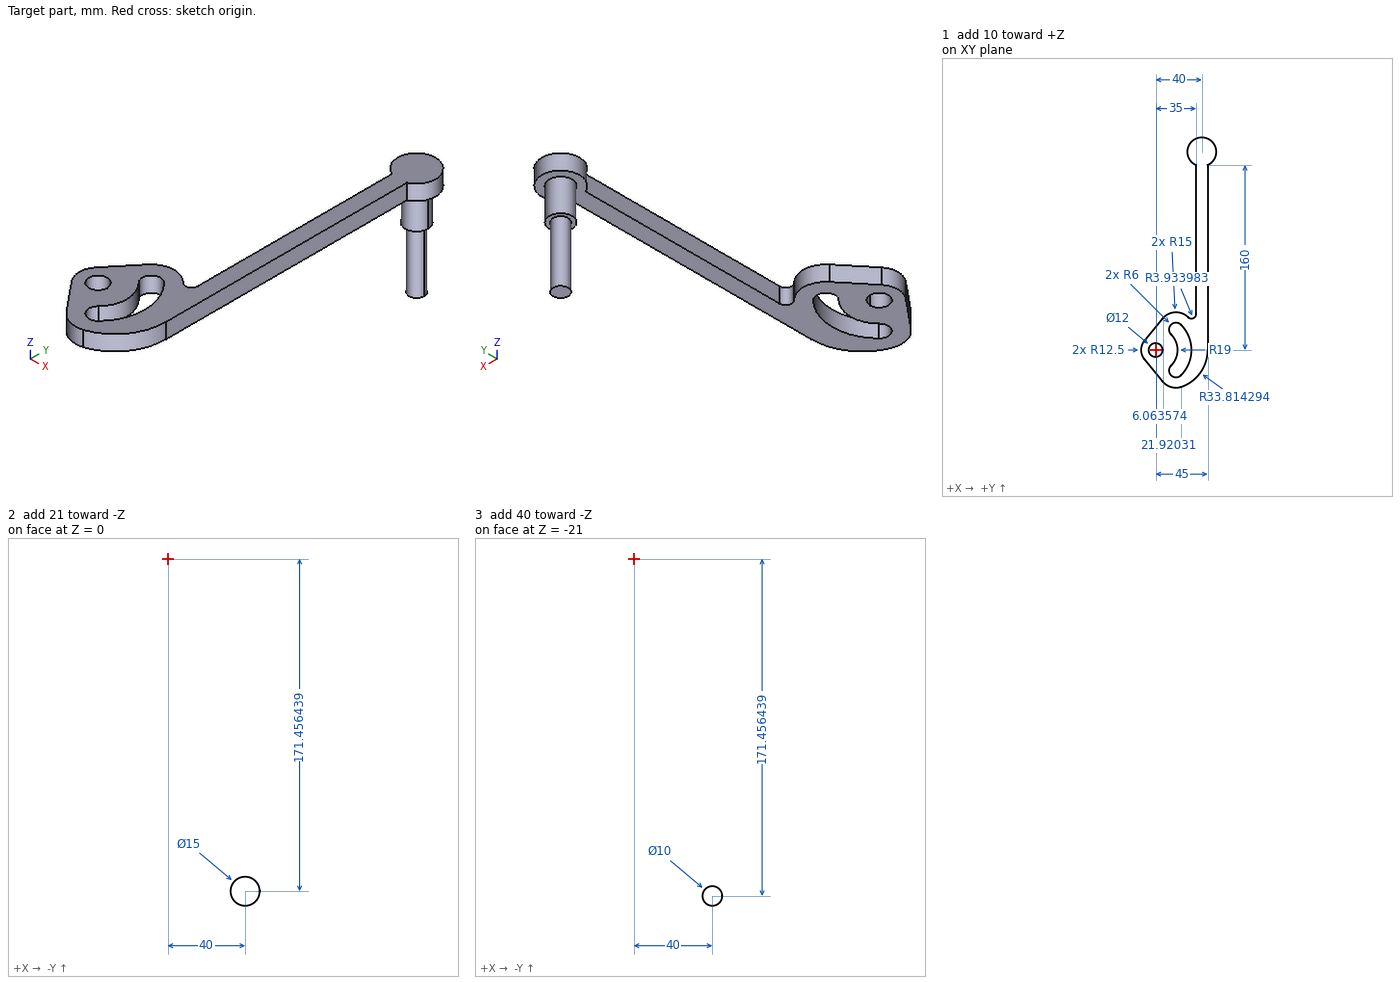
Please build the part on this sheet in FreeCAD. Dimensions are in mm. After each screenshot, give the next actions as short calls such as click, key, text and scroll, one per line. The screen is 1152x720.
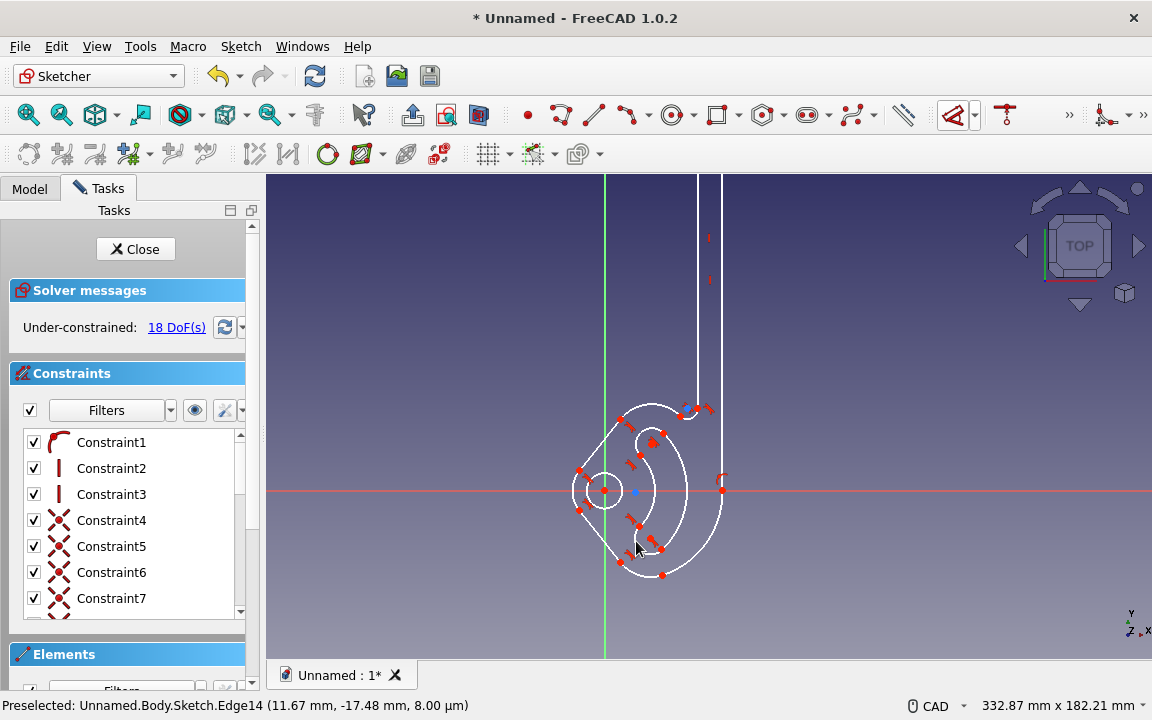
scroll(605, 491, up, 7)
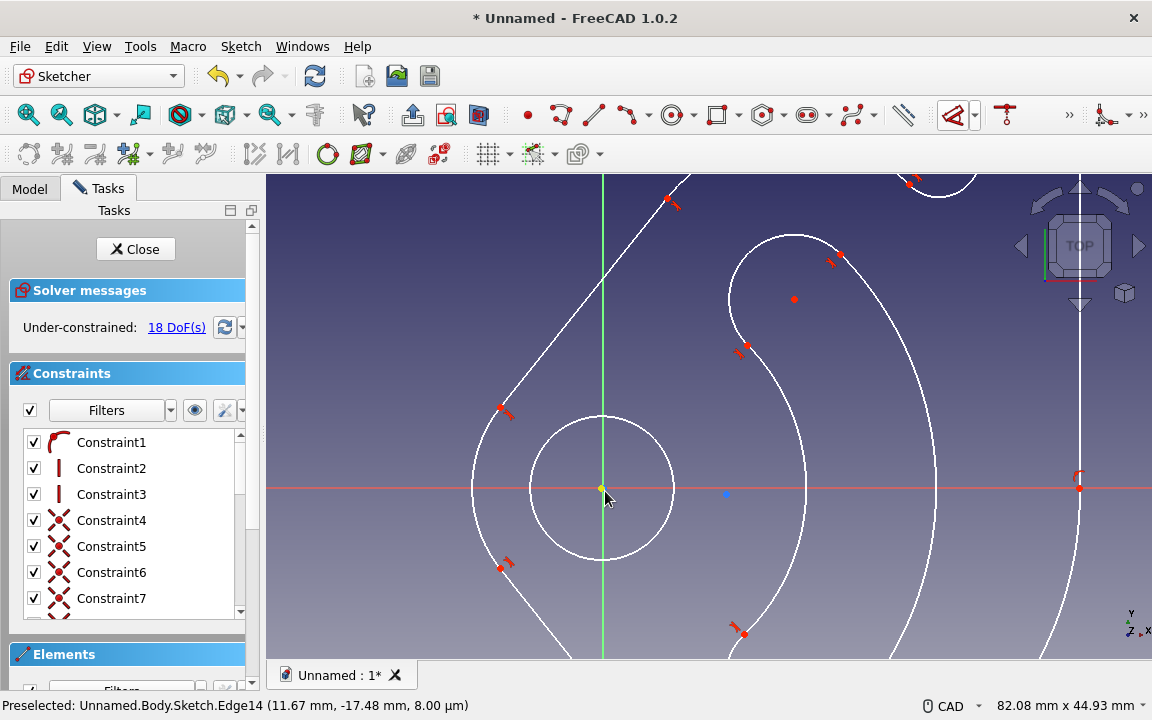
drag(592, 478, 613, 498)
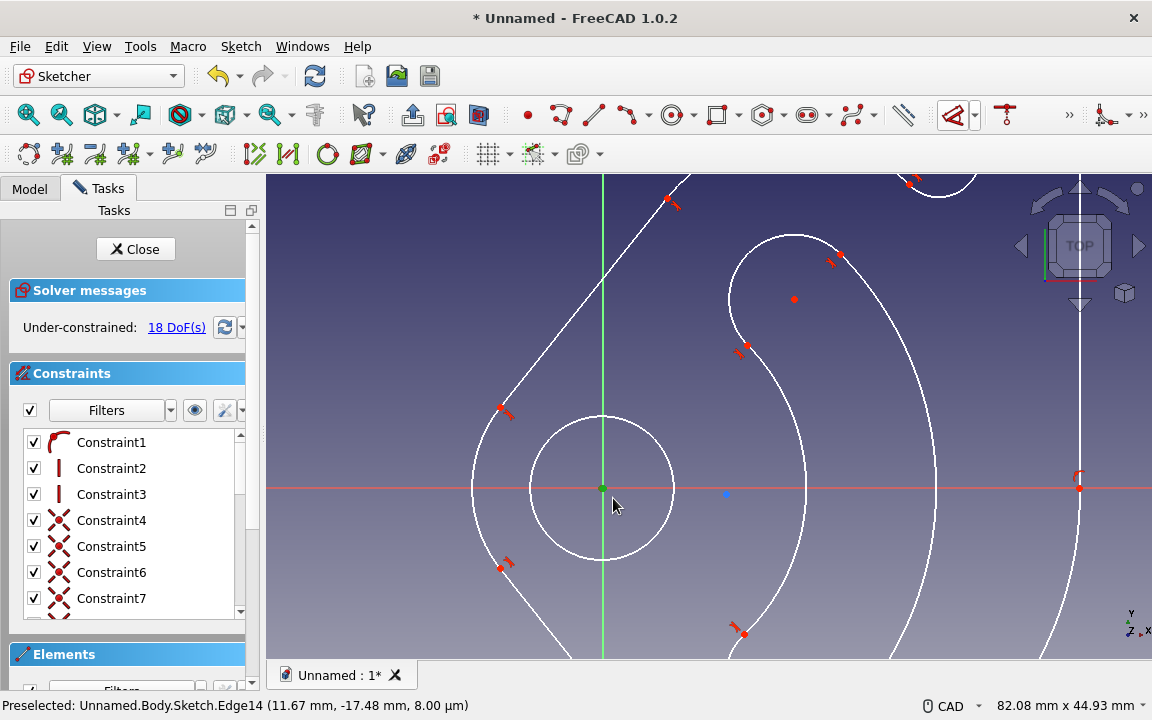
click(1005, 116)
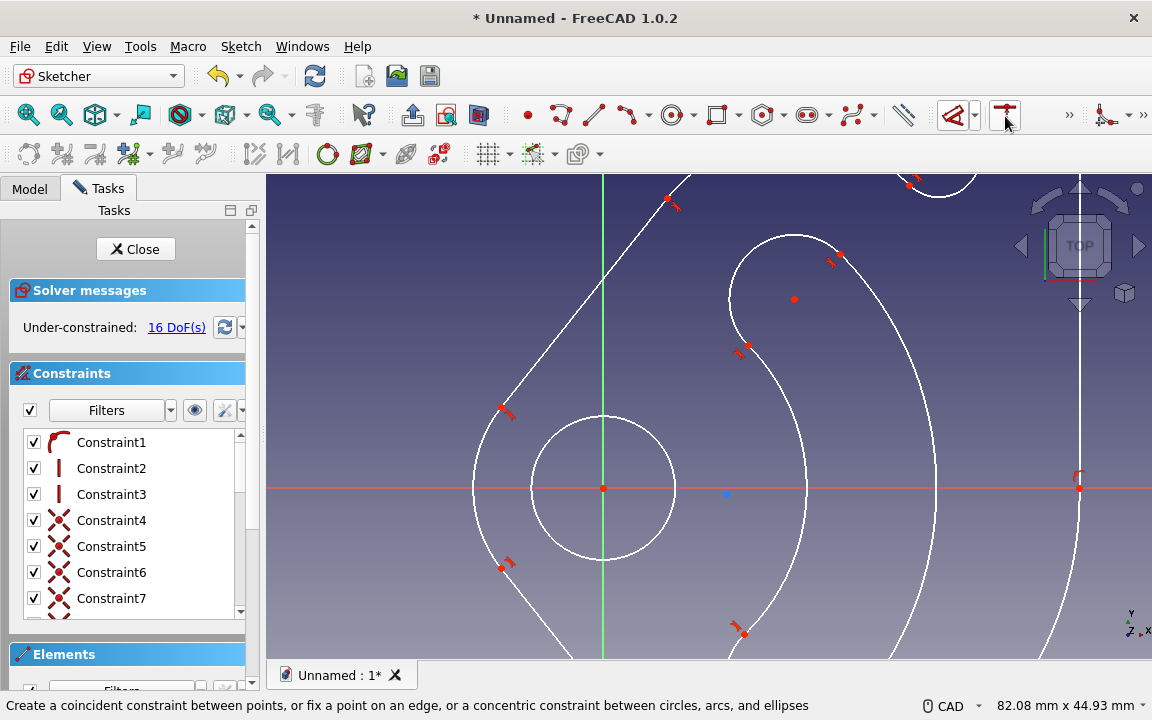
click(478, 454)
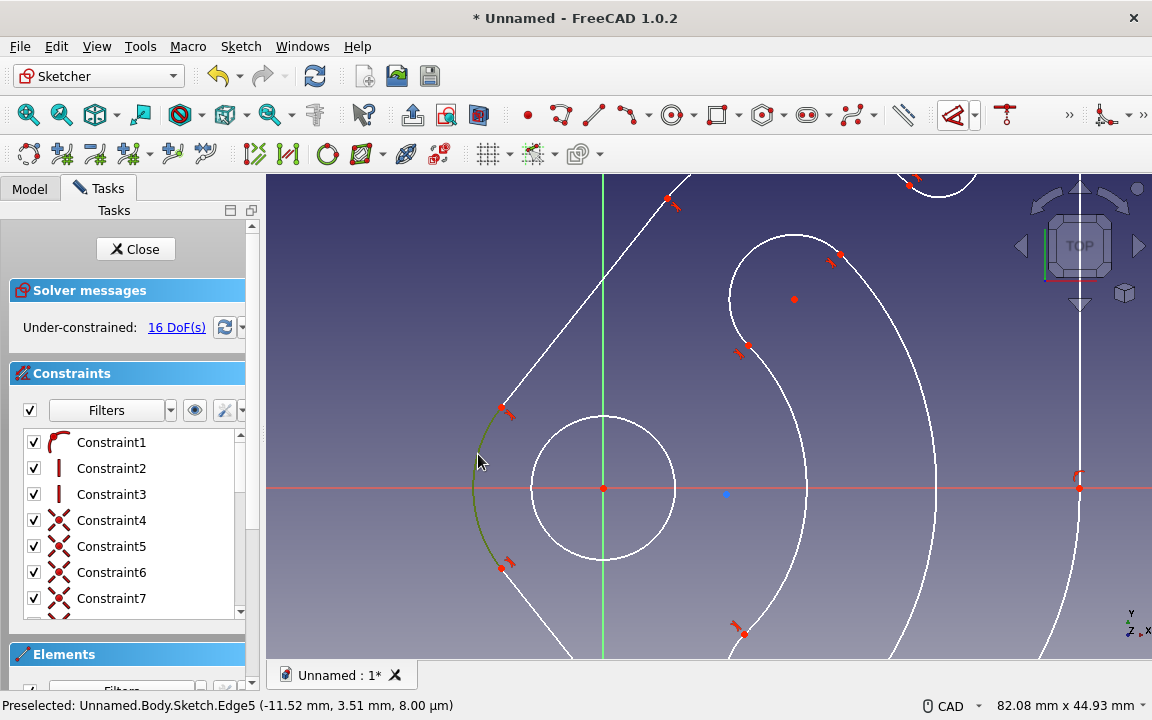
scroll(619, 534, down, 10)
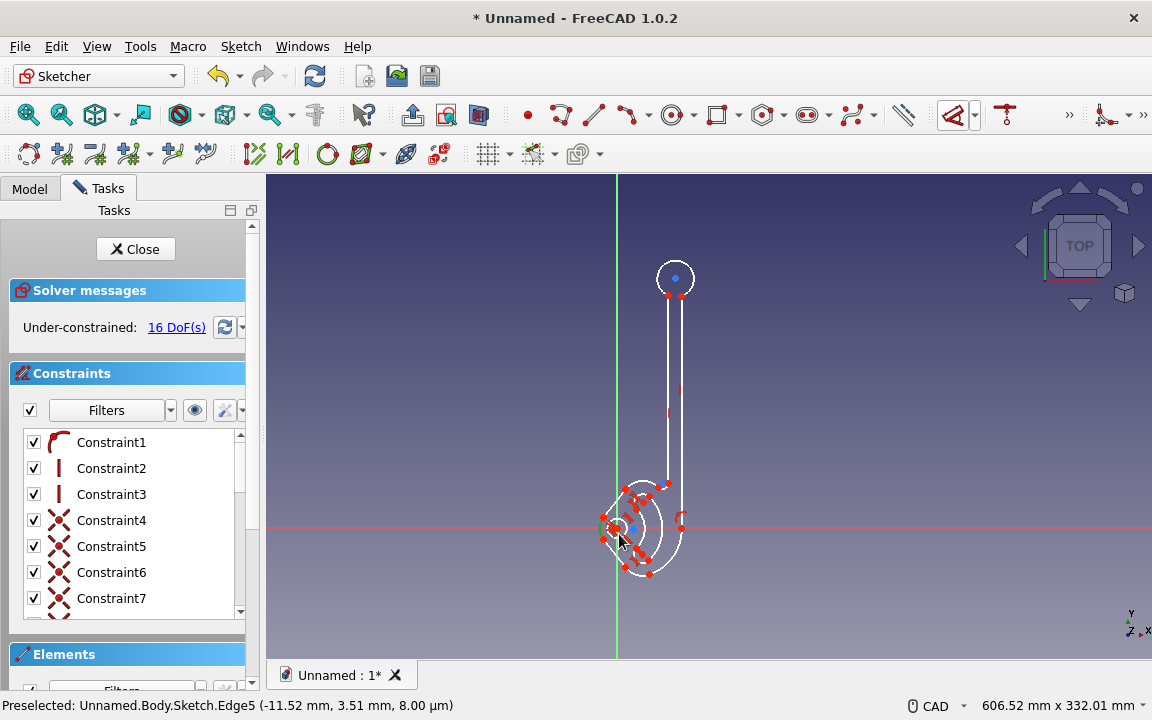
click(692, 271)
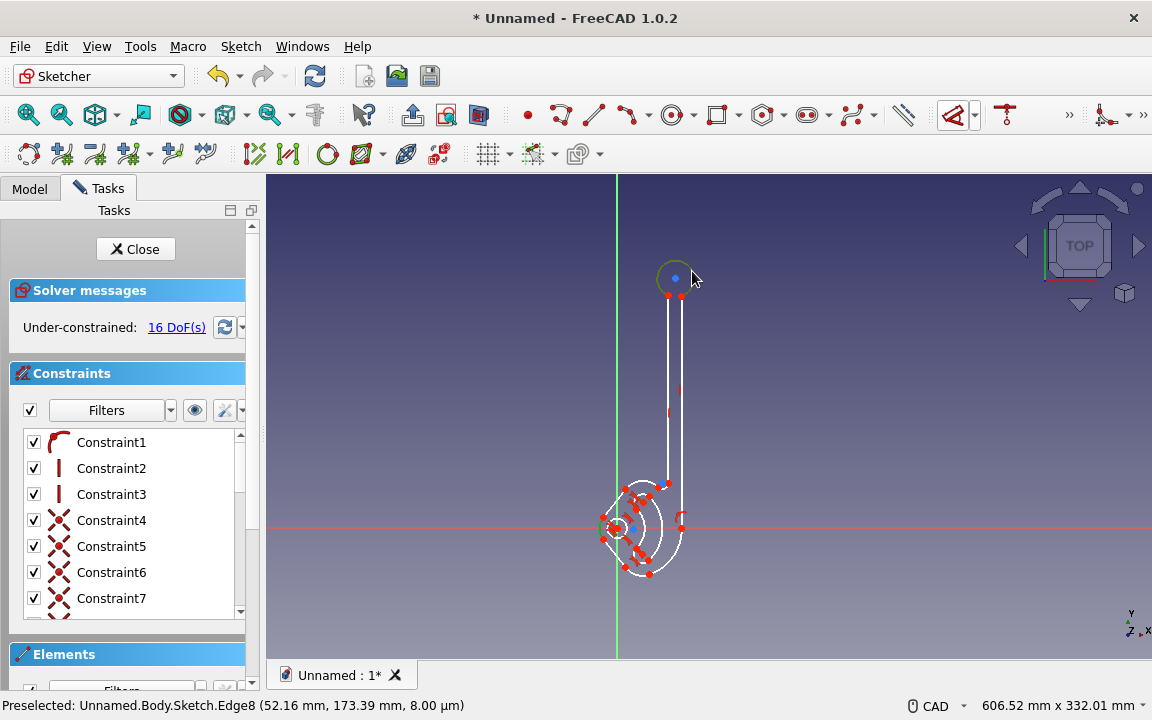
key(e)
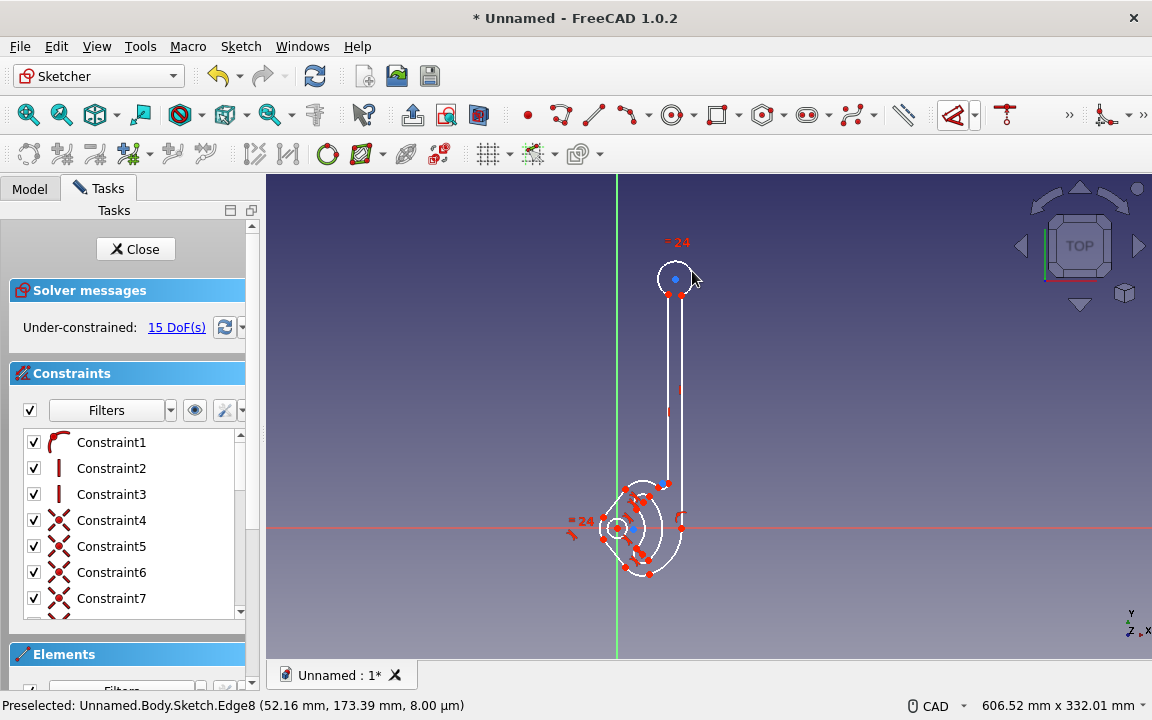
click(636, 575)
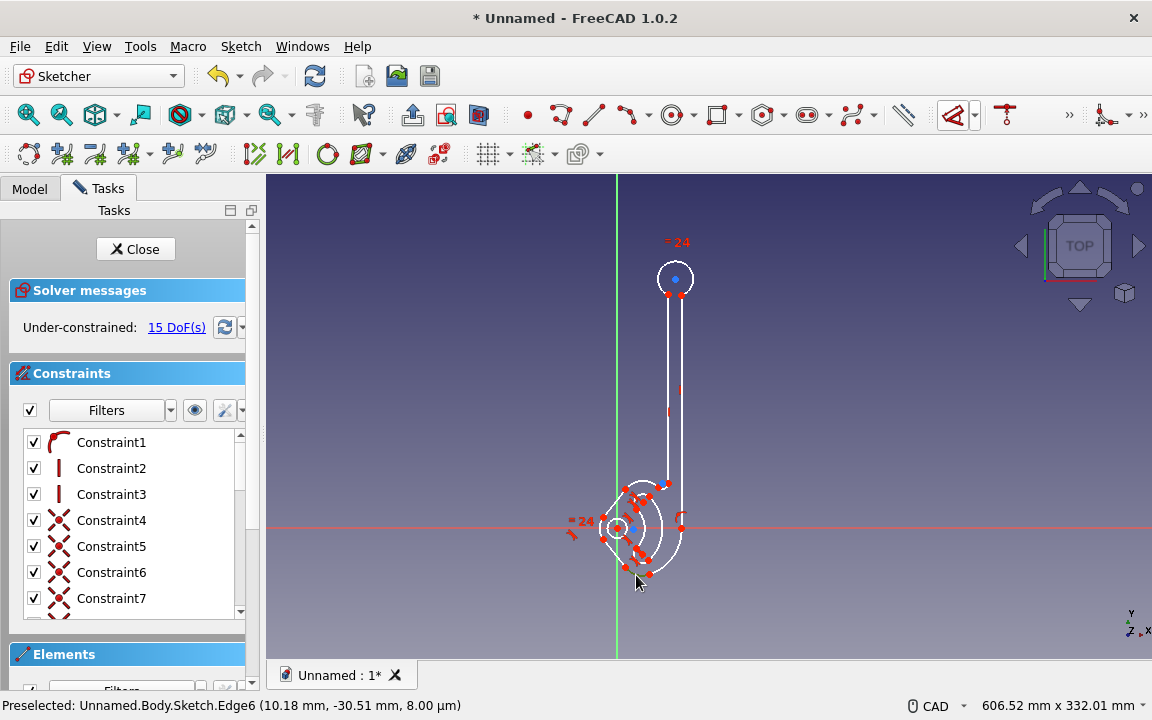
scroll(649, 482, up, 2)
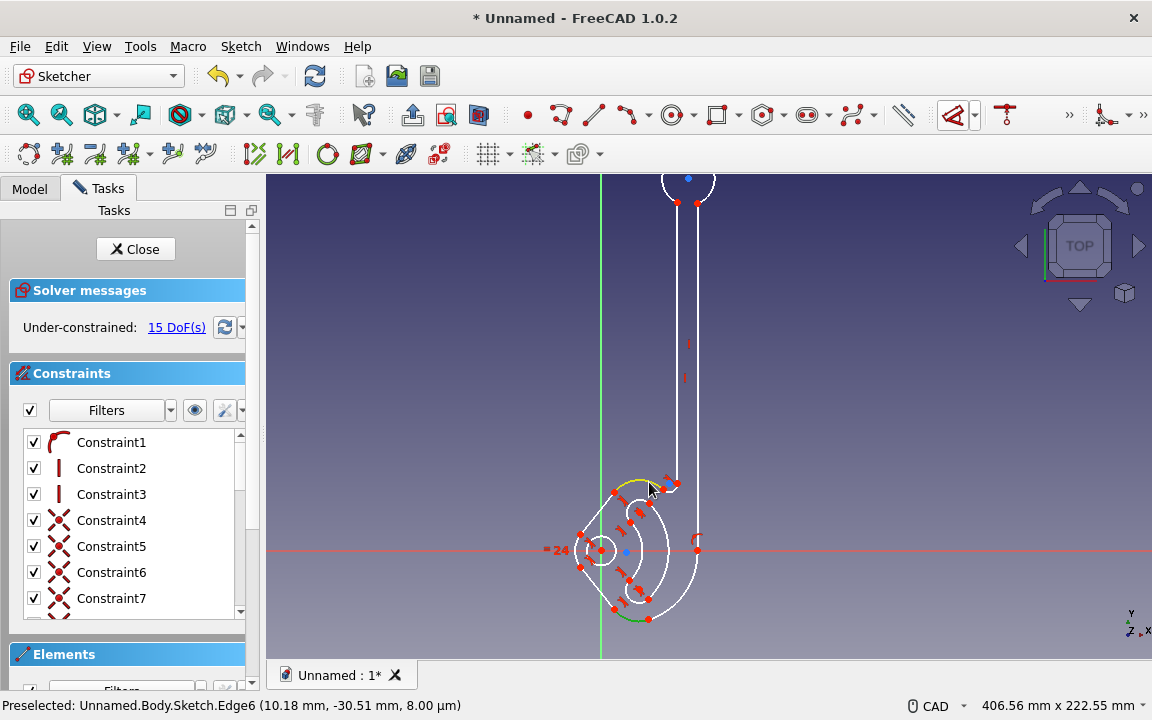
click(649, 481)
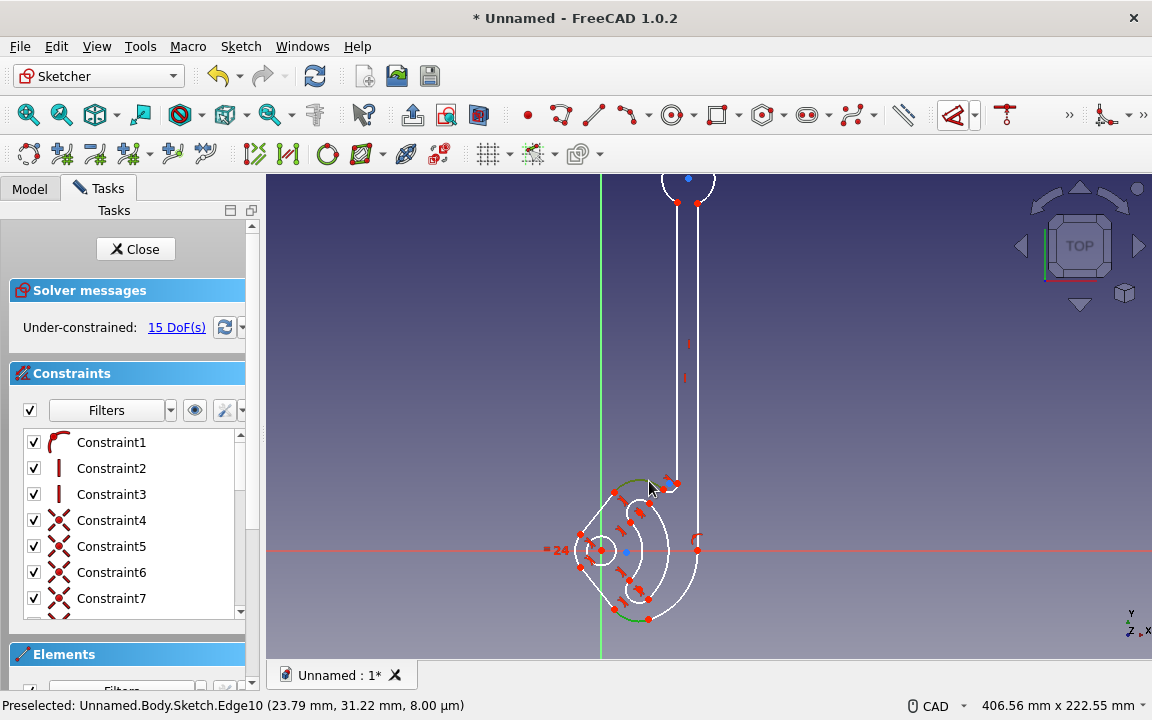
key(e)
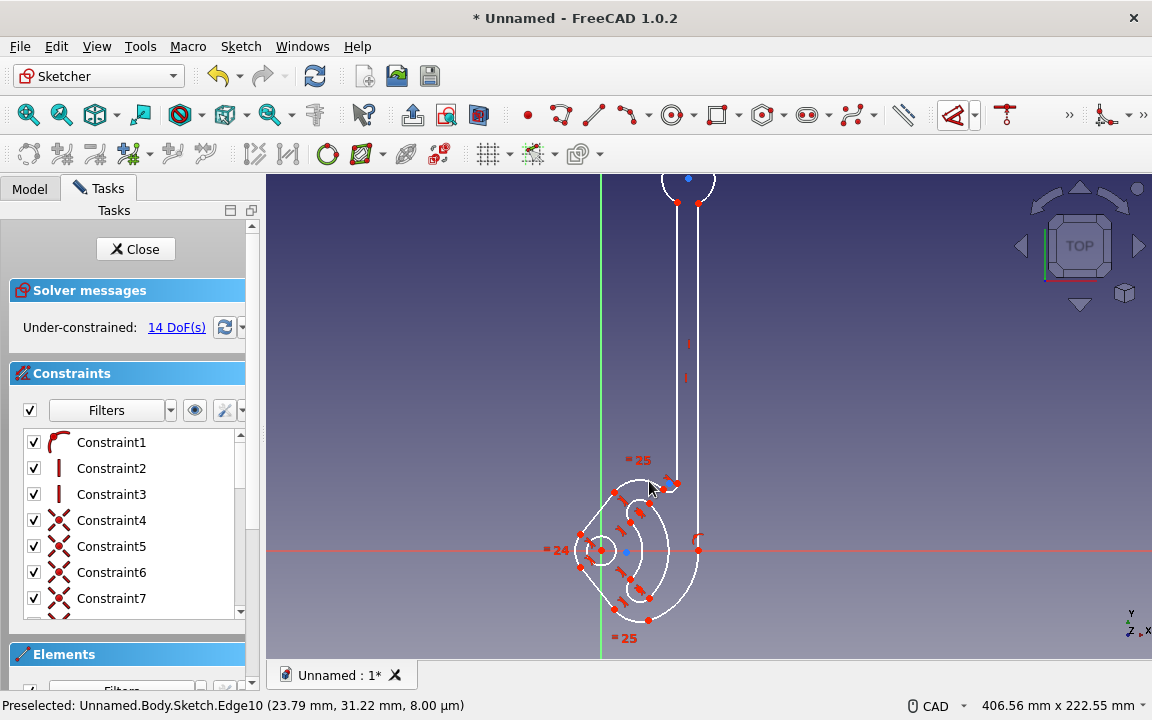
click(626, 552)